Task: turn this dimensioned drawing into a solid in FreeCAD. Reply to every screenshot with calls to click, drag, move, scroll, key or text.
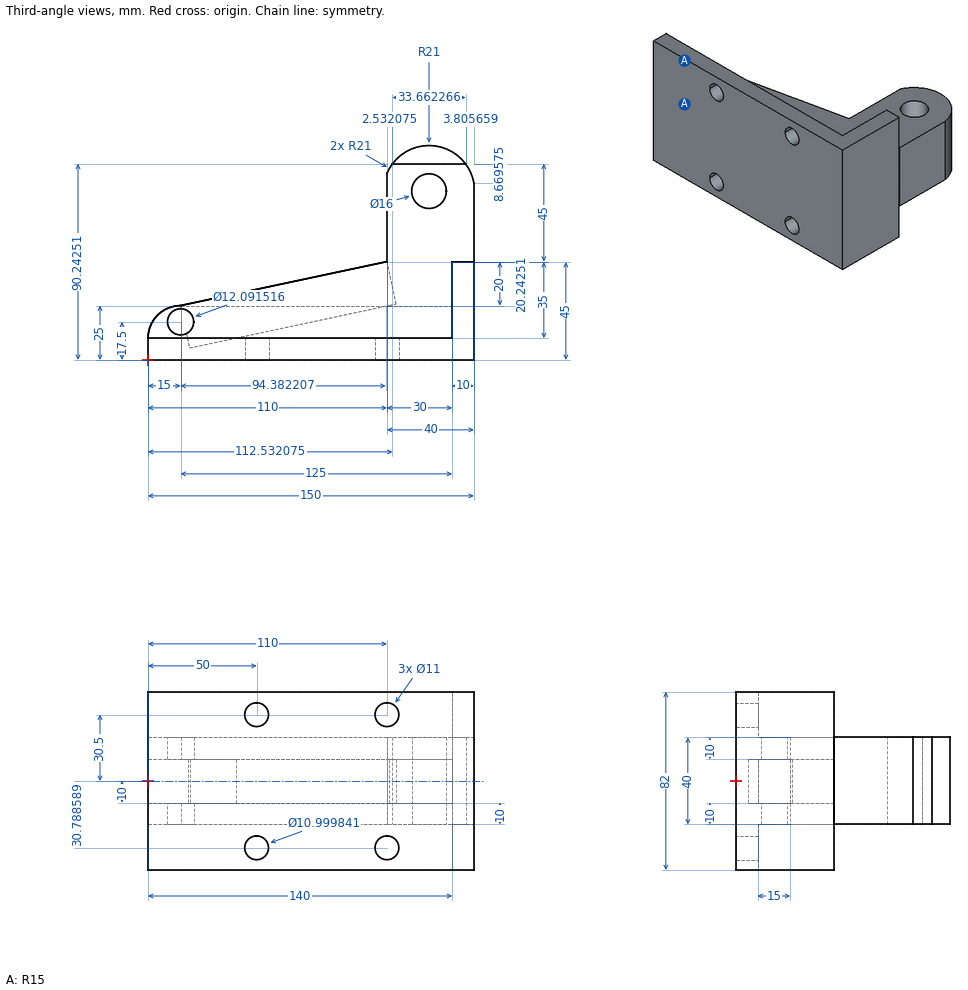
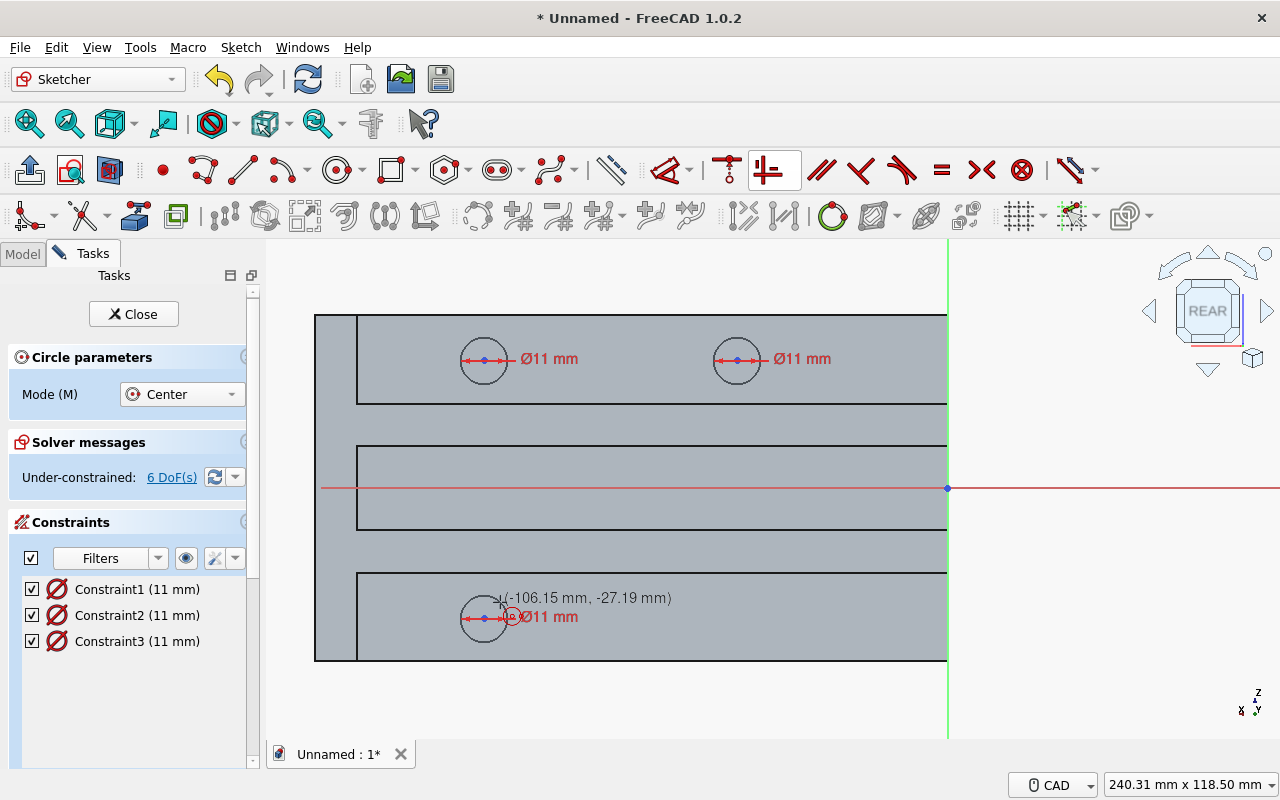
click(737, 618)
move(753, 602)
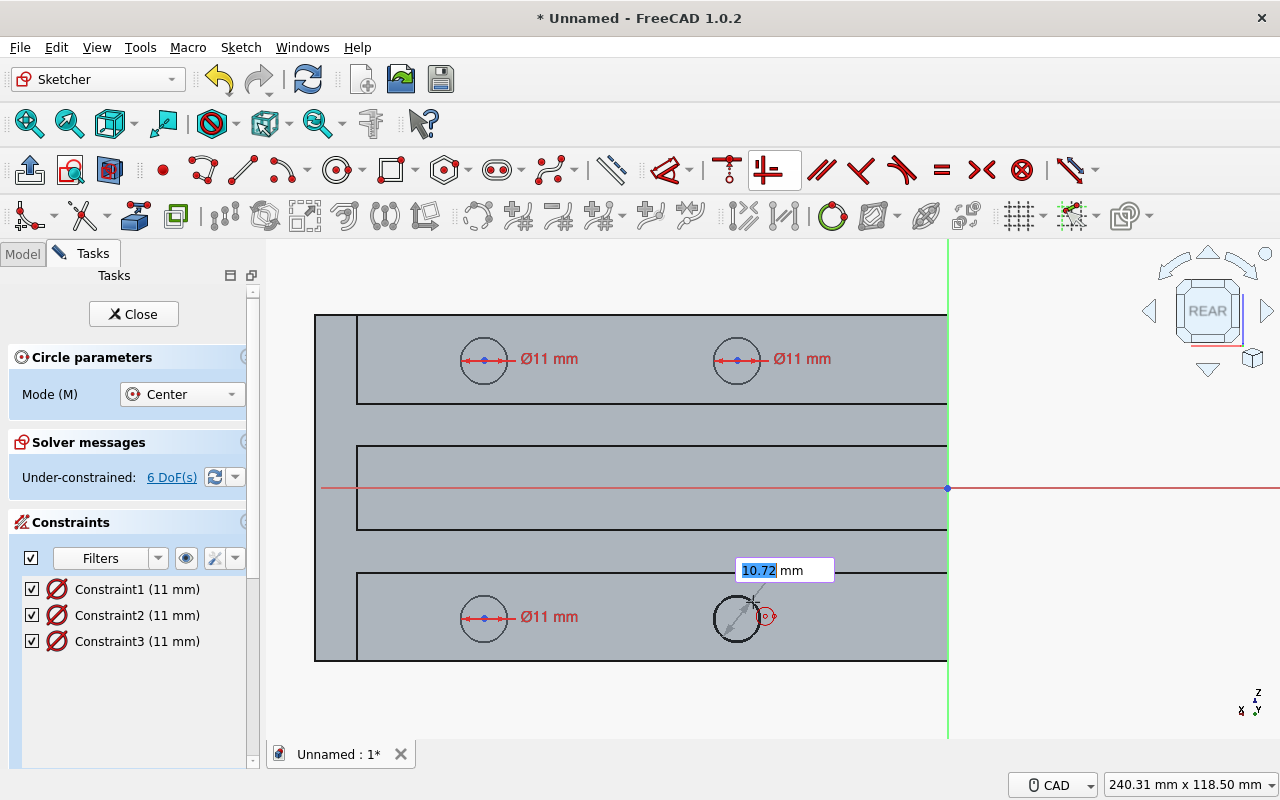
text(10.999841)
key(Return)
key(Escape)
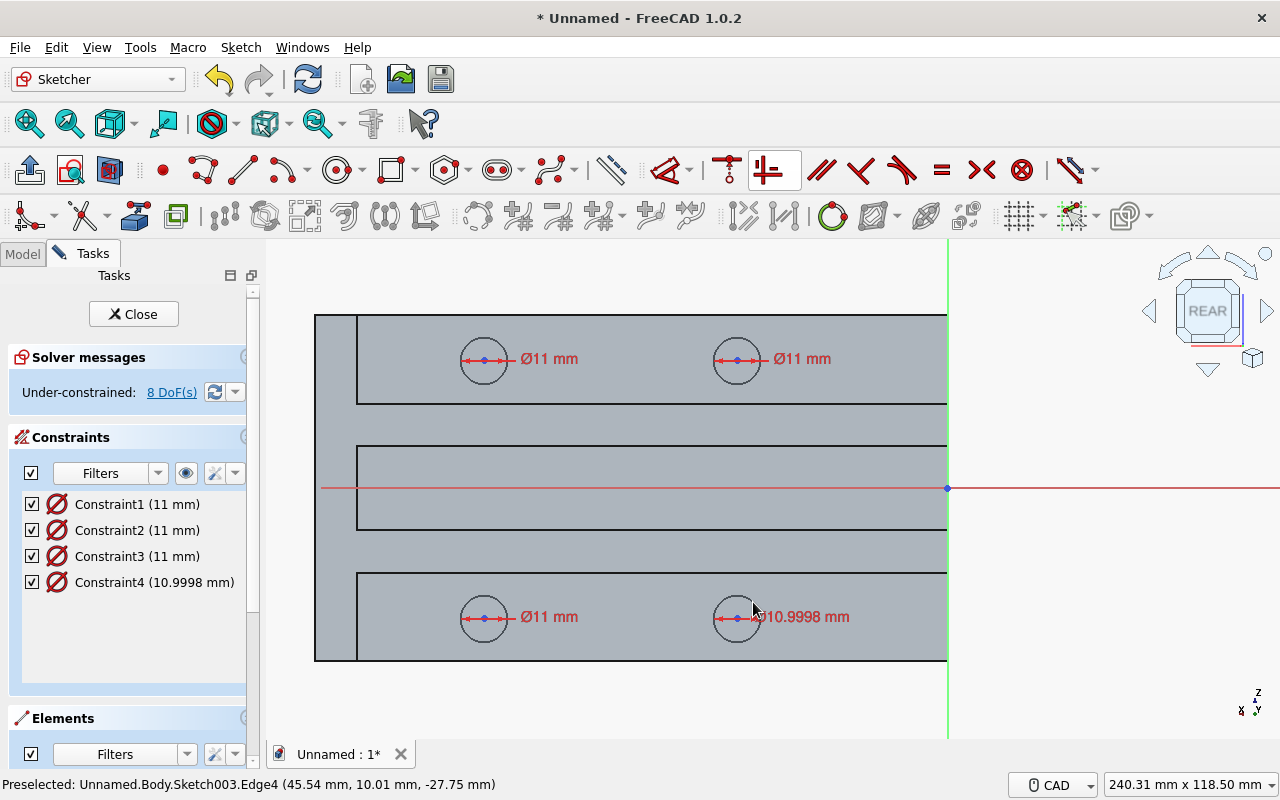
click(484, 361)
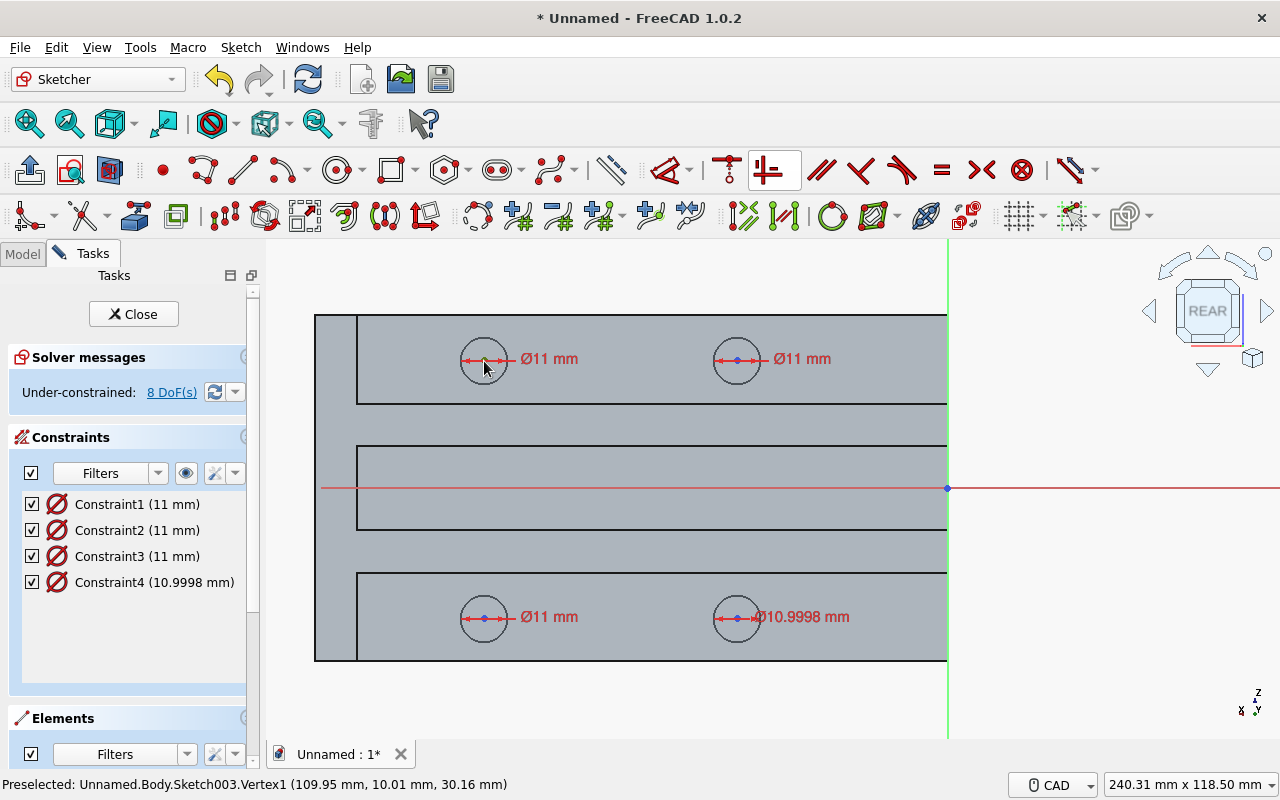
click(737, 361)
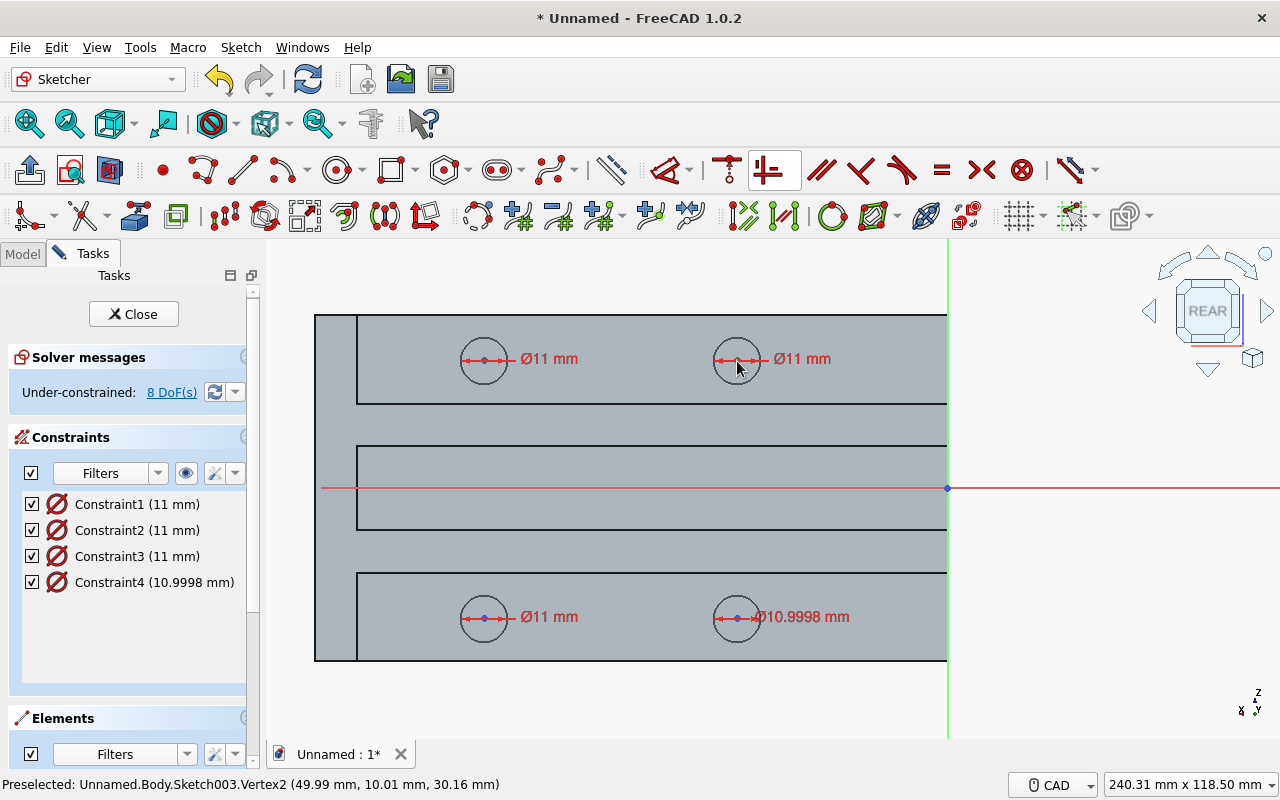
key(h)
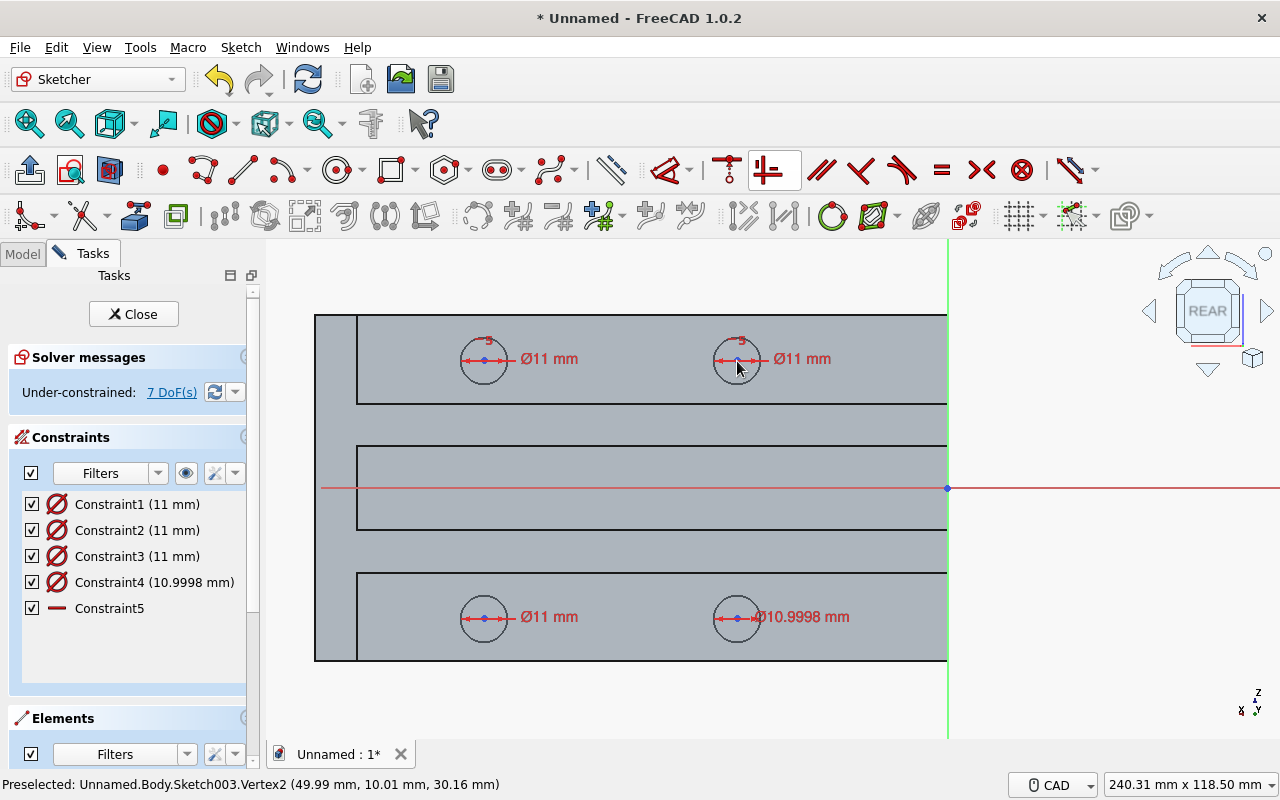
click(484, 361)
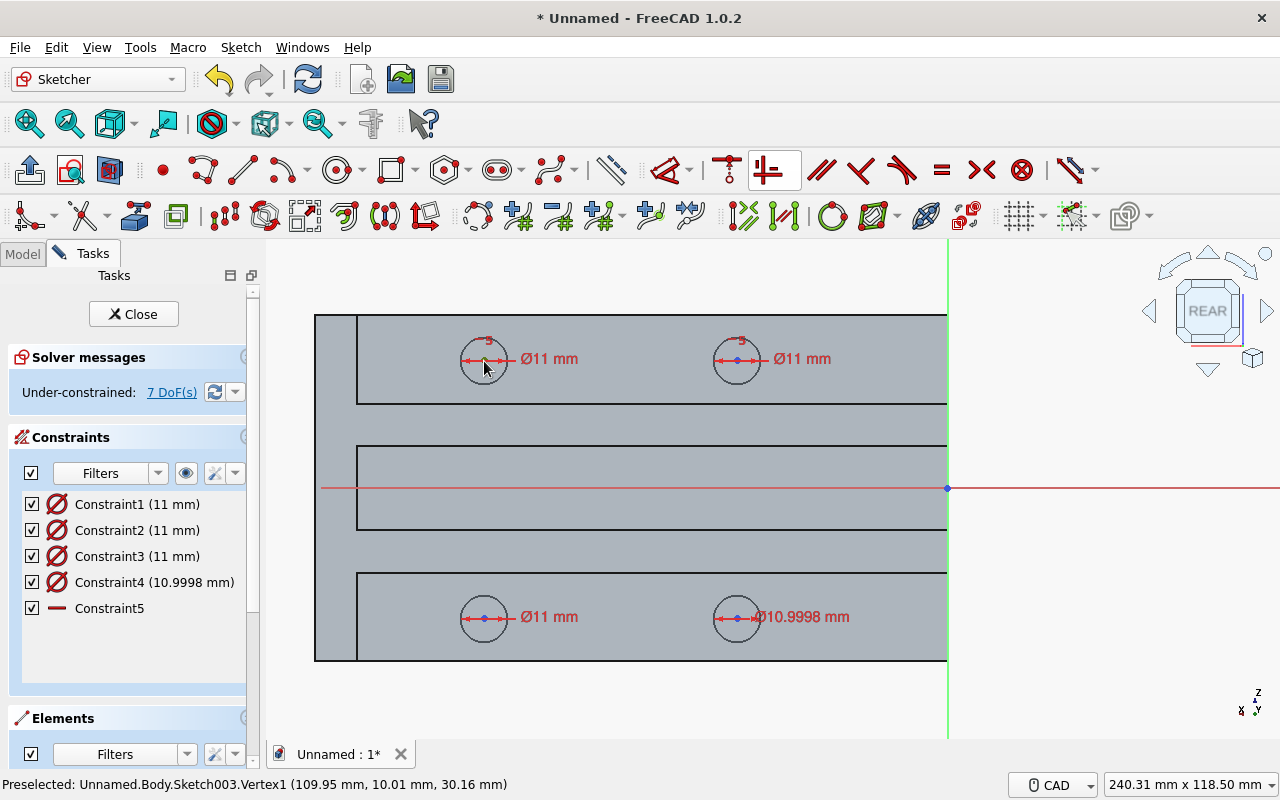
click(484, 619)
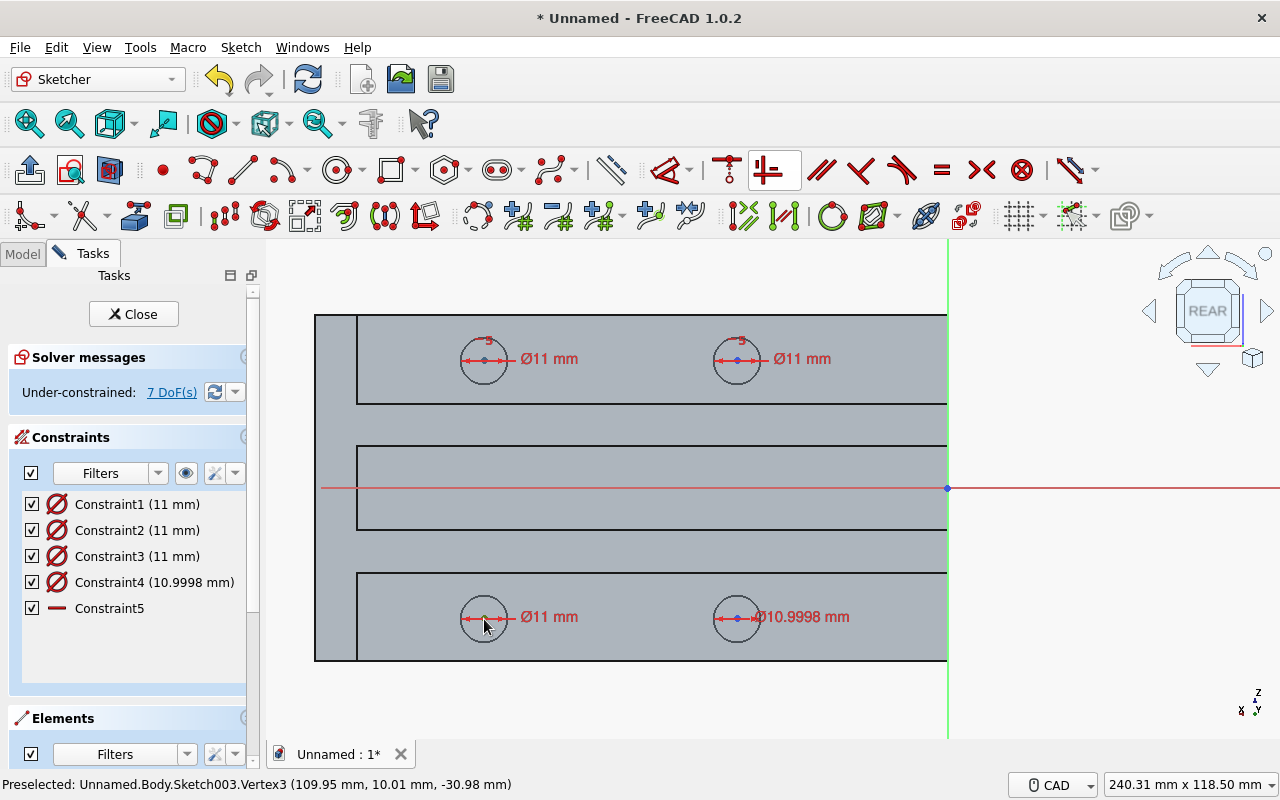
key(v)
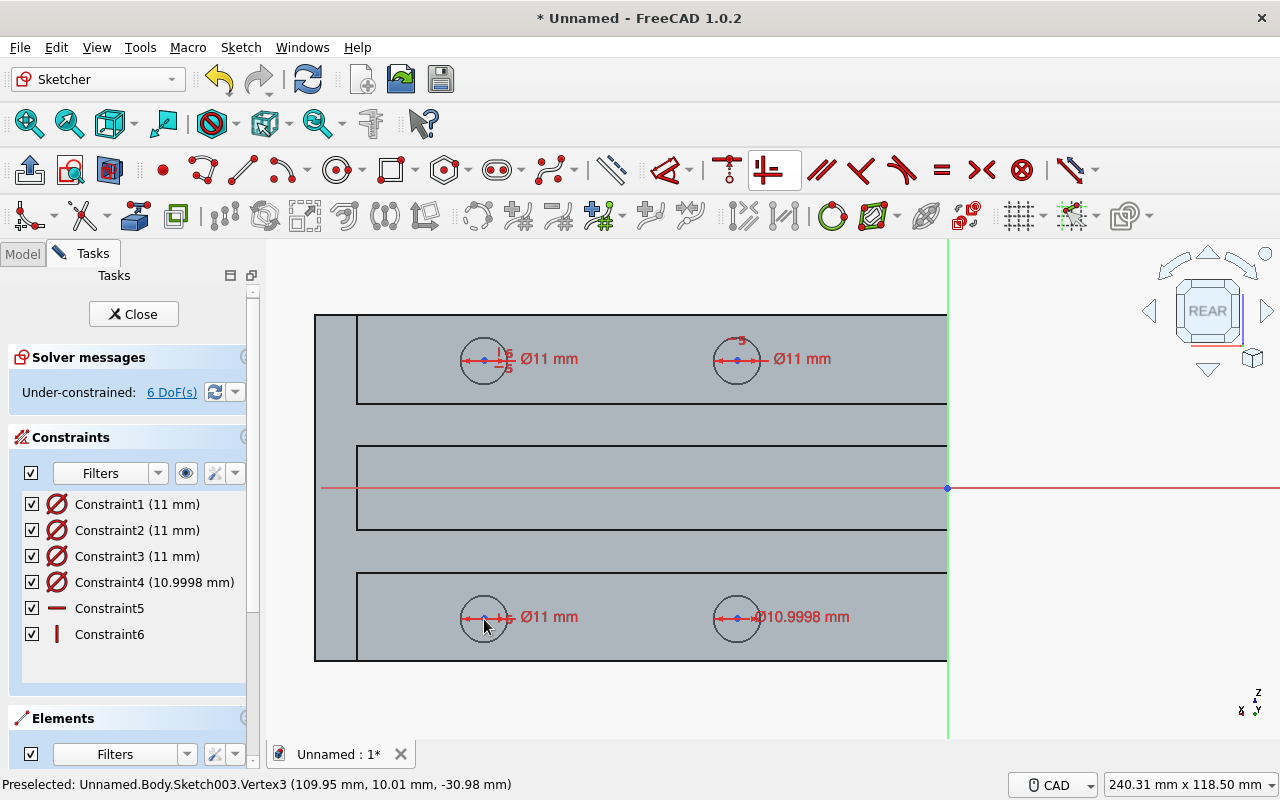
click(737, 361)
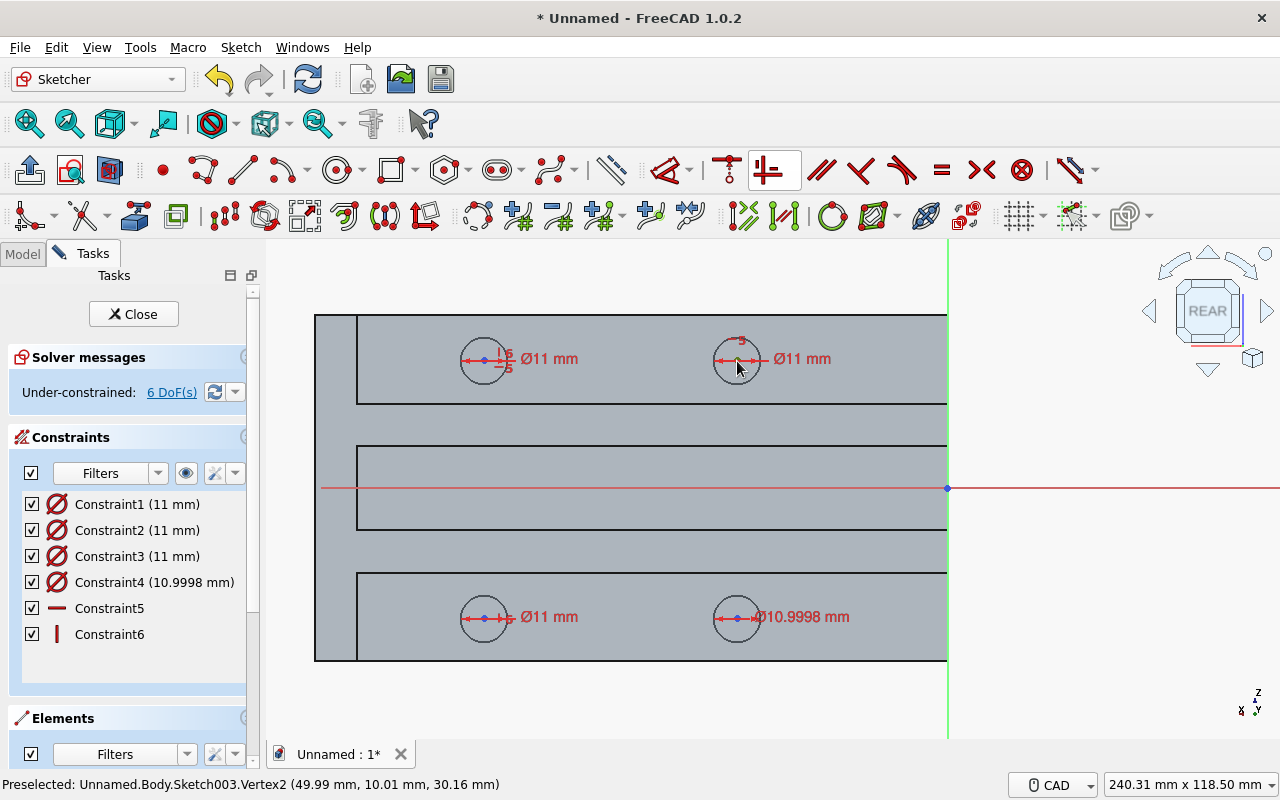
click(737, 619)